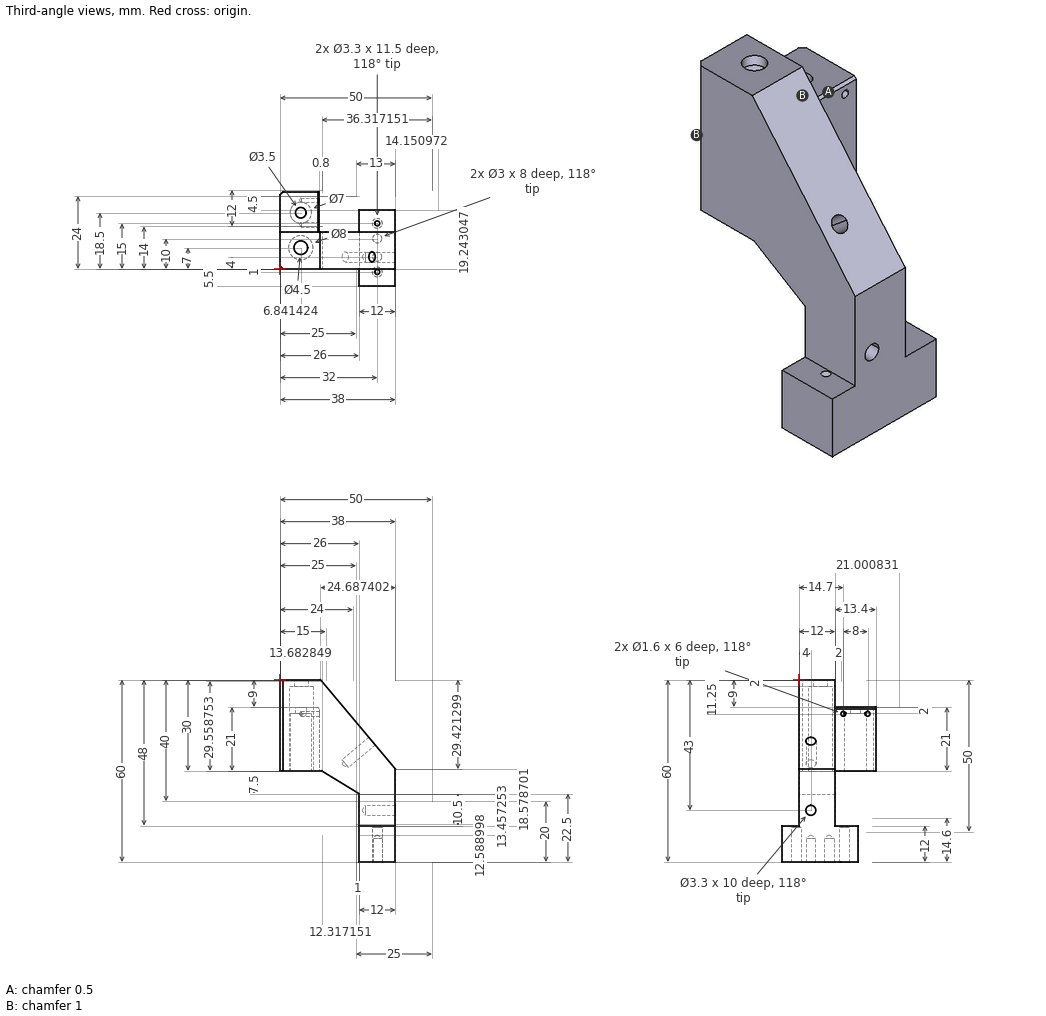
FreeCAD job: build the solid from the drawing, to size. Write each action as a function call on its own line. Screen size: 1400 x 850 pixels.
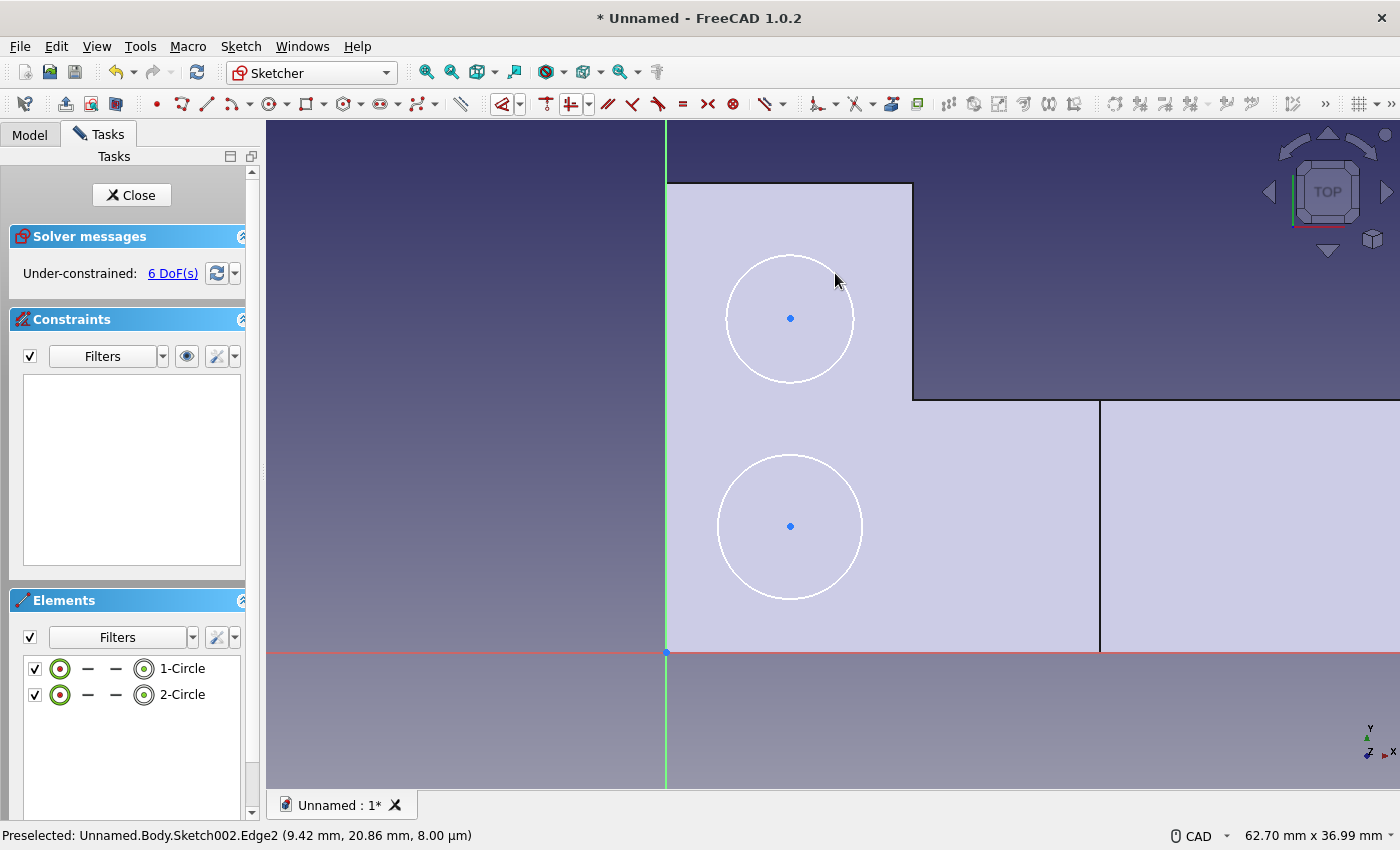
click(790, 527)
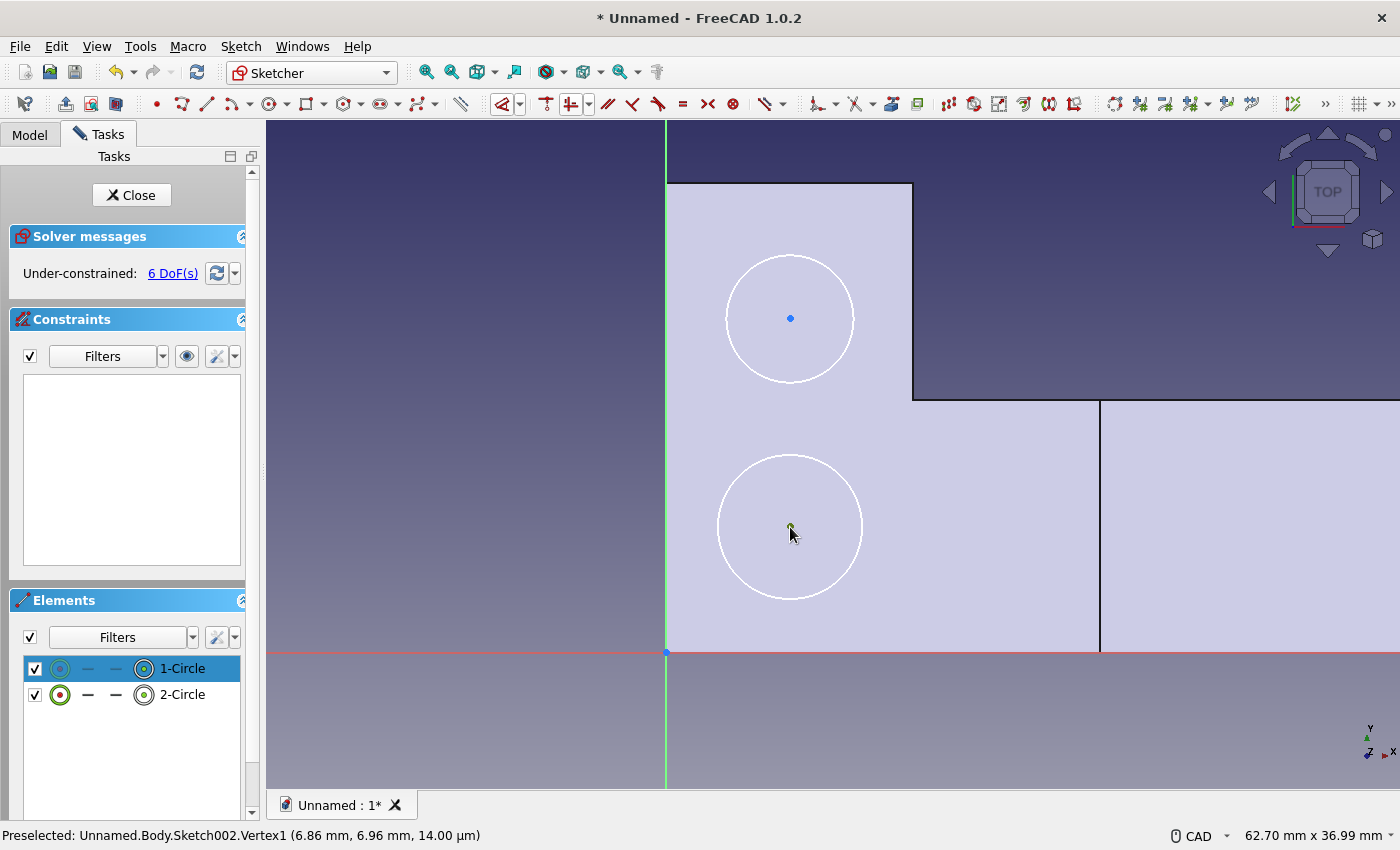
click(790, 319)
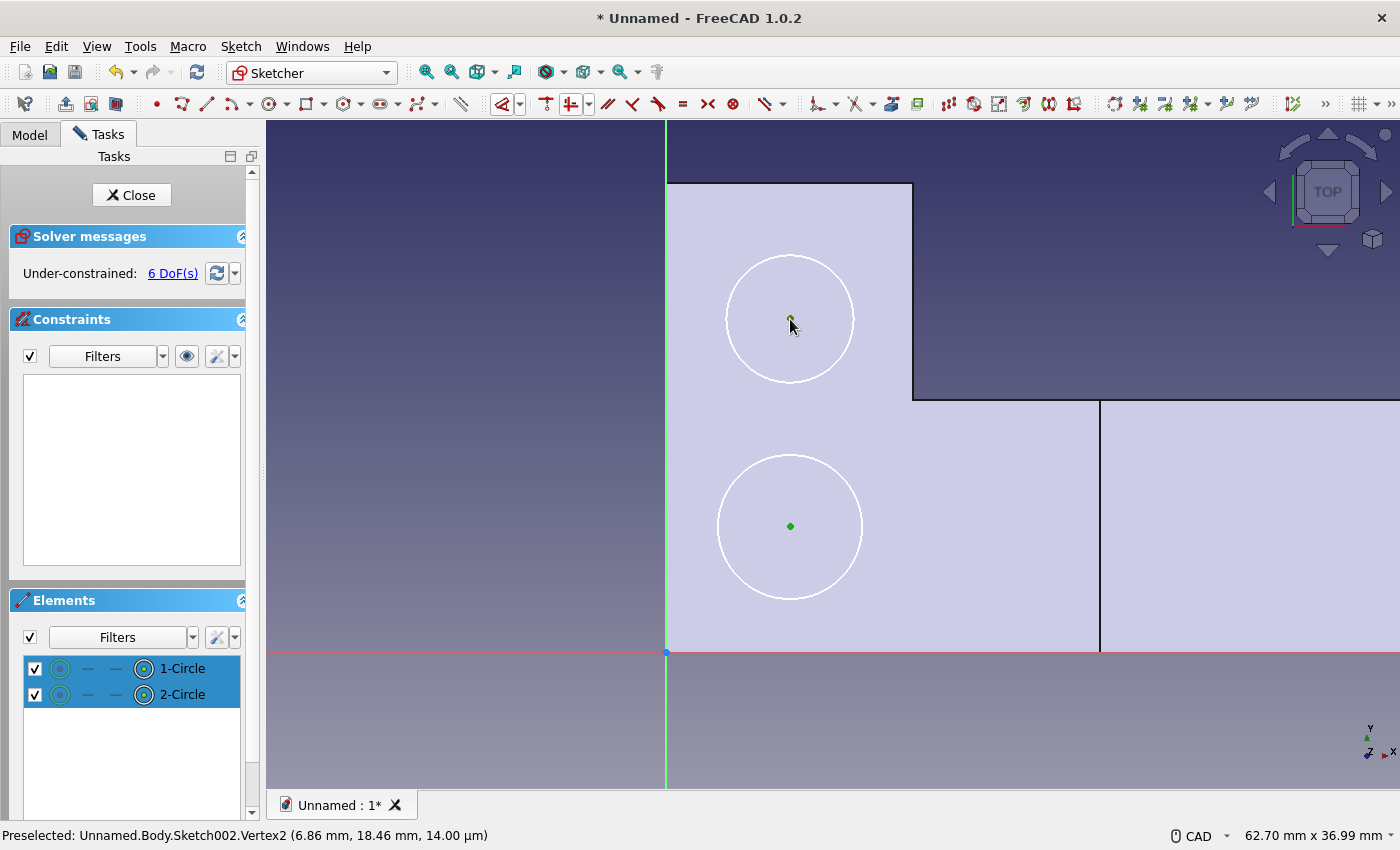
key(v)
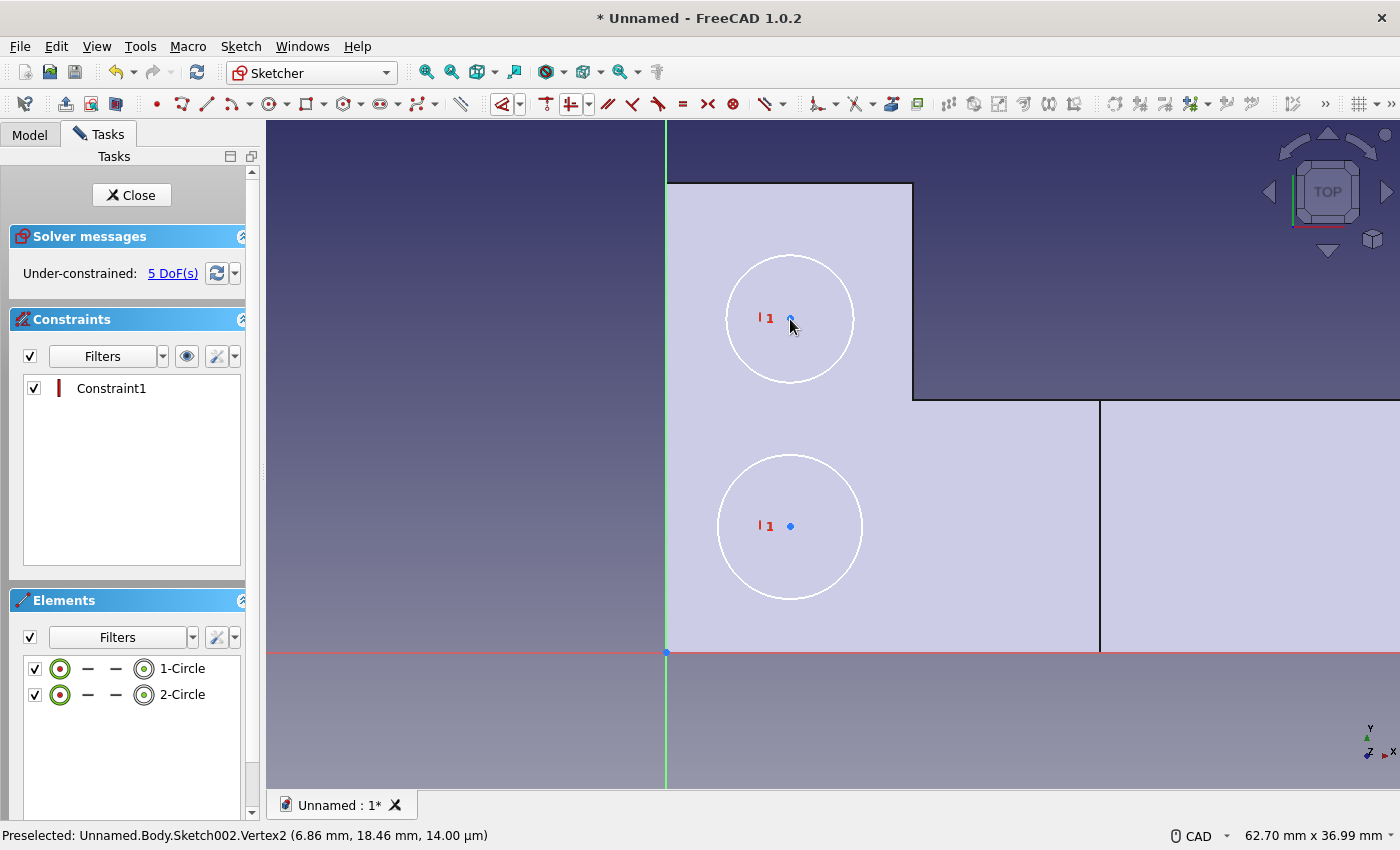
click(841, 476)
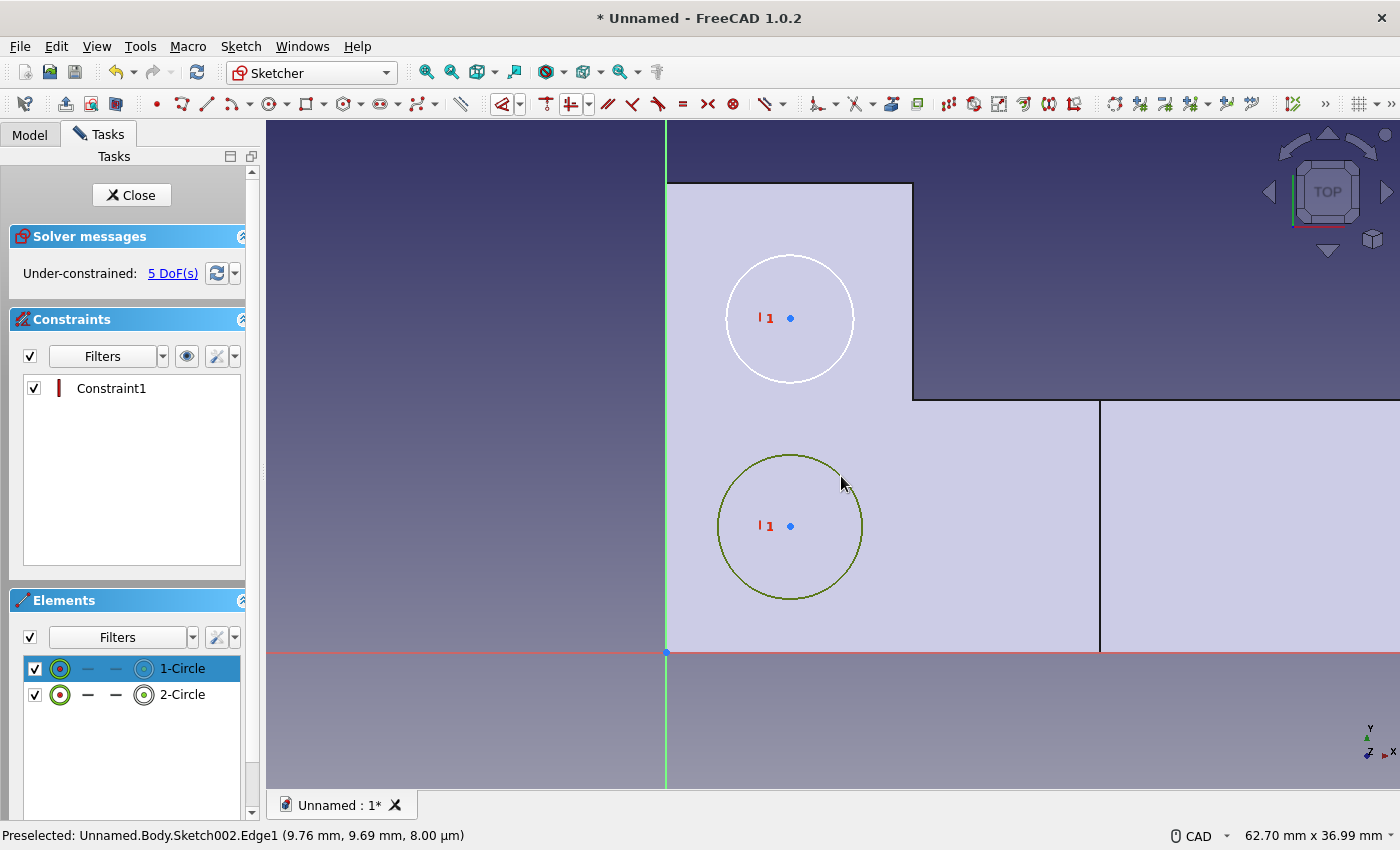
click(520, 104)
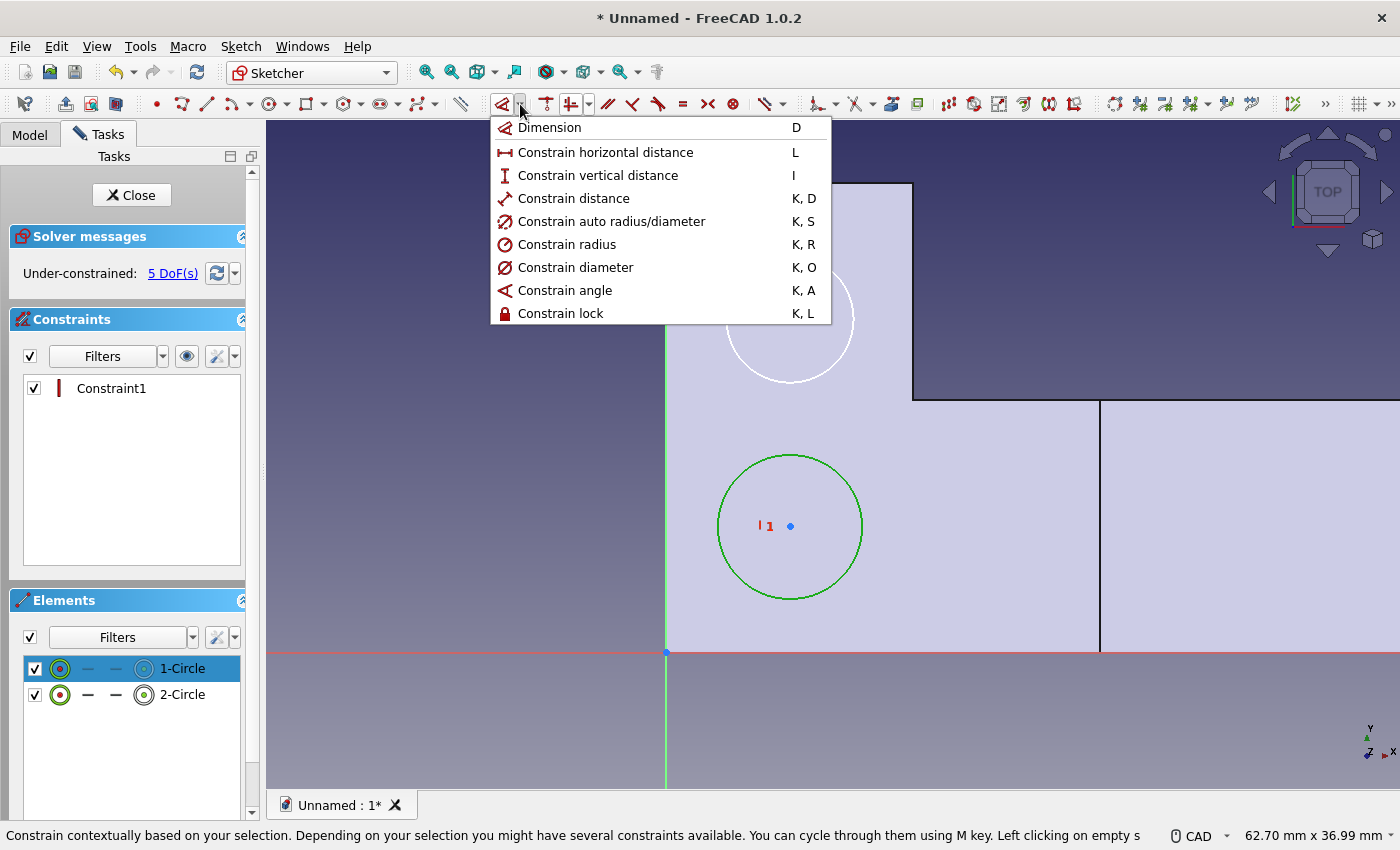
click(661, 268)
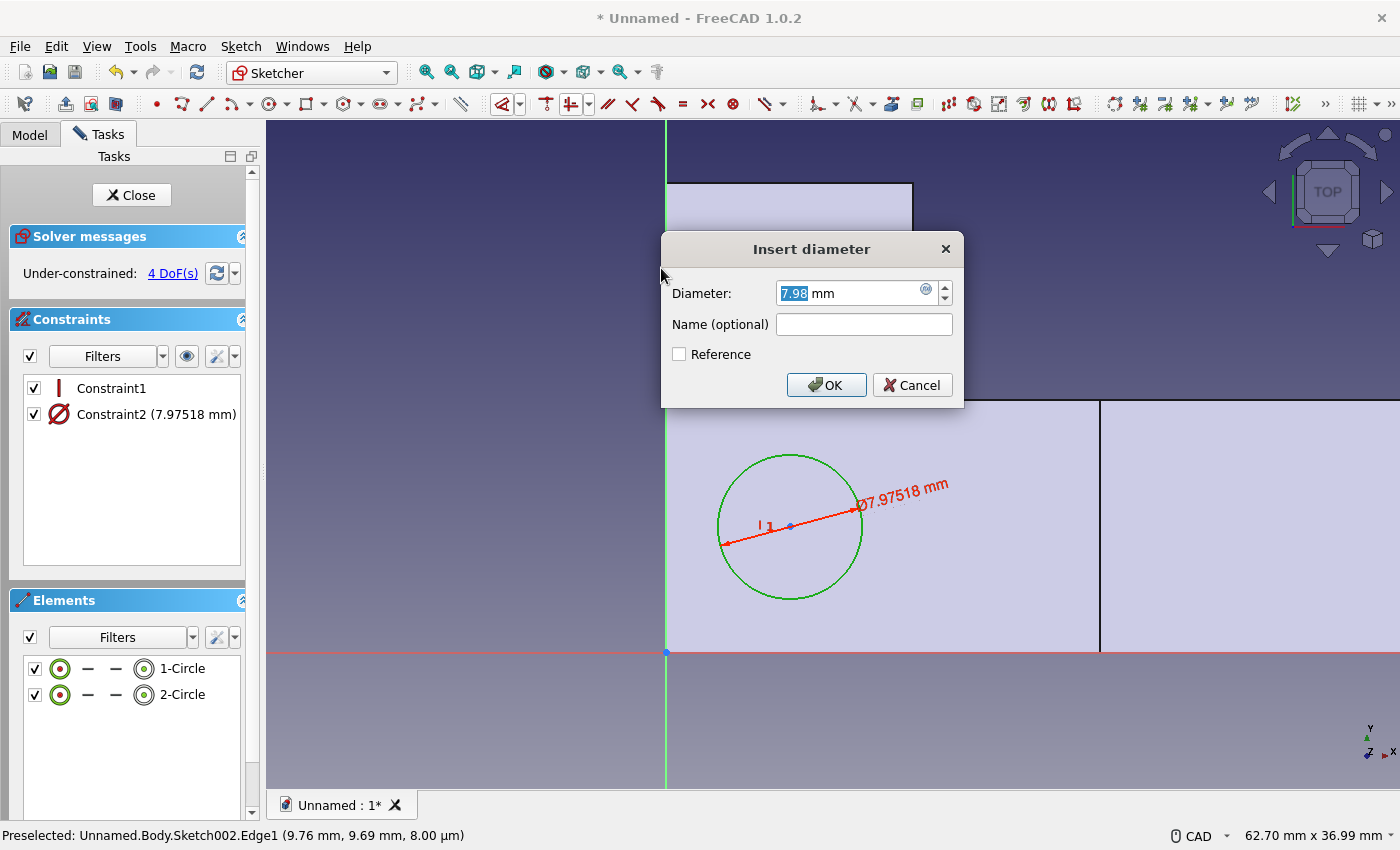
text(8)
key(Return)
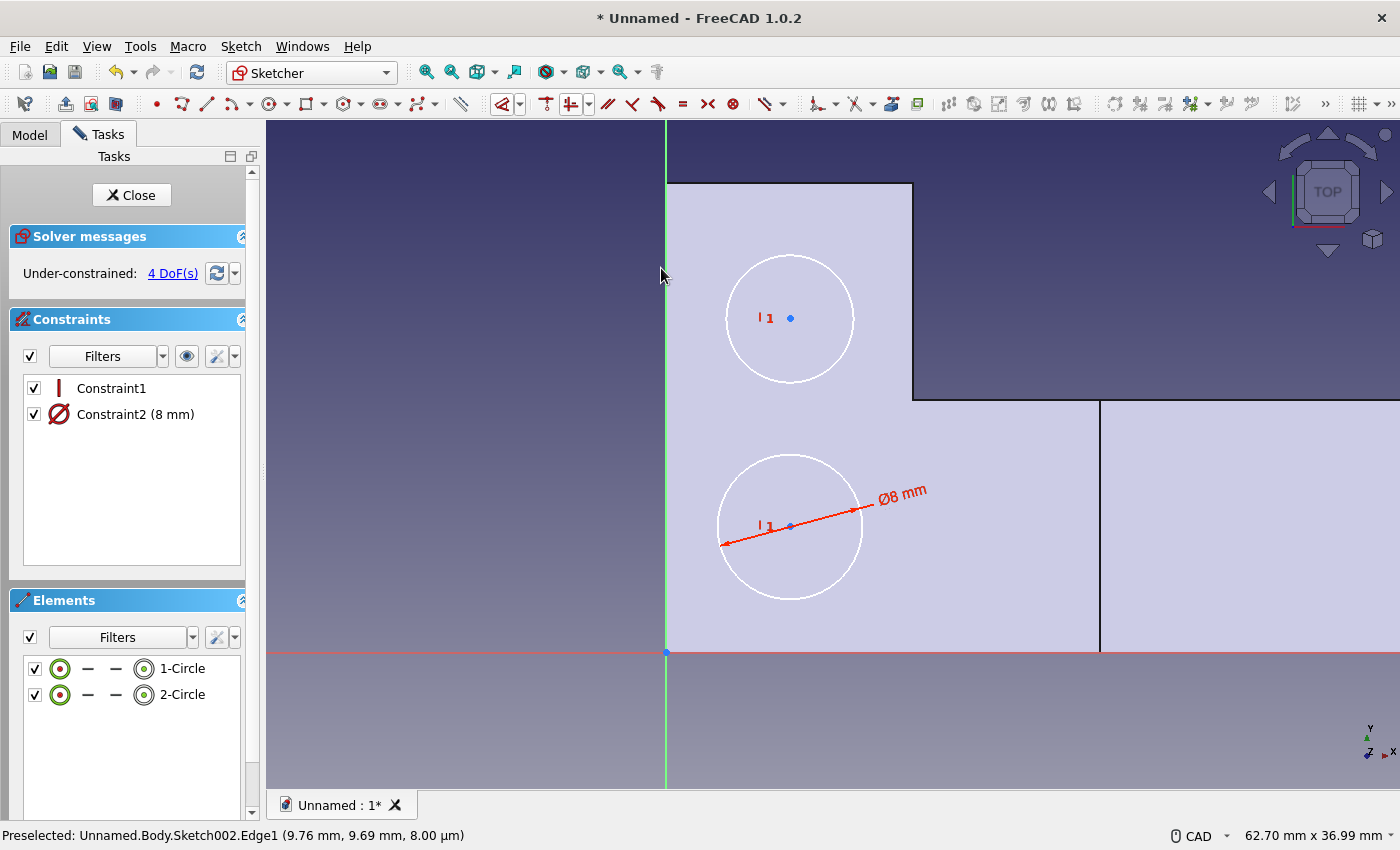
click(835, 274)